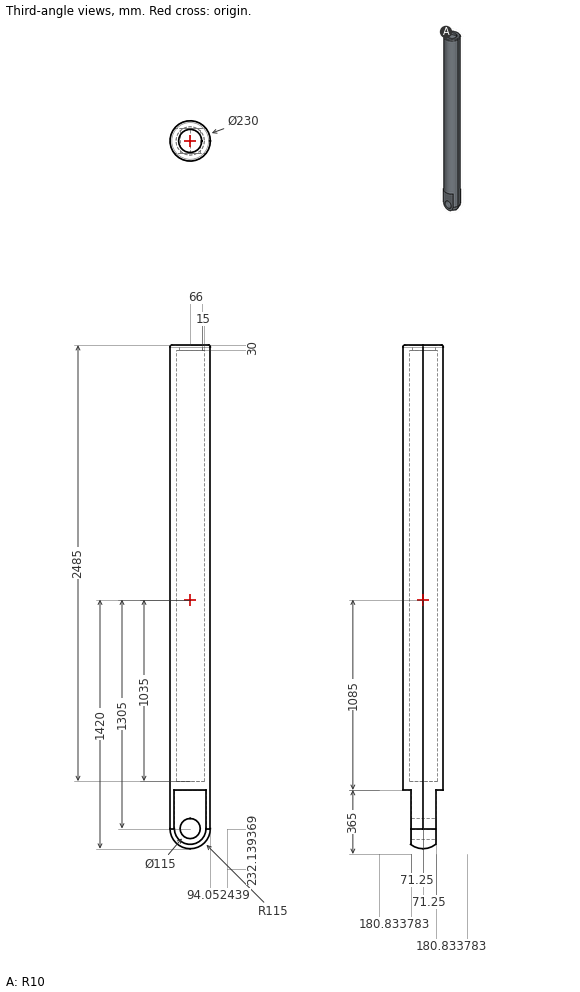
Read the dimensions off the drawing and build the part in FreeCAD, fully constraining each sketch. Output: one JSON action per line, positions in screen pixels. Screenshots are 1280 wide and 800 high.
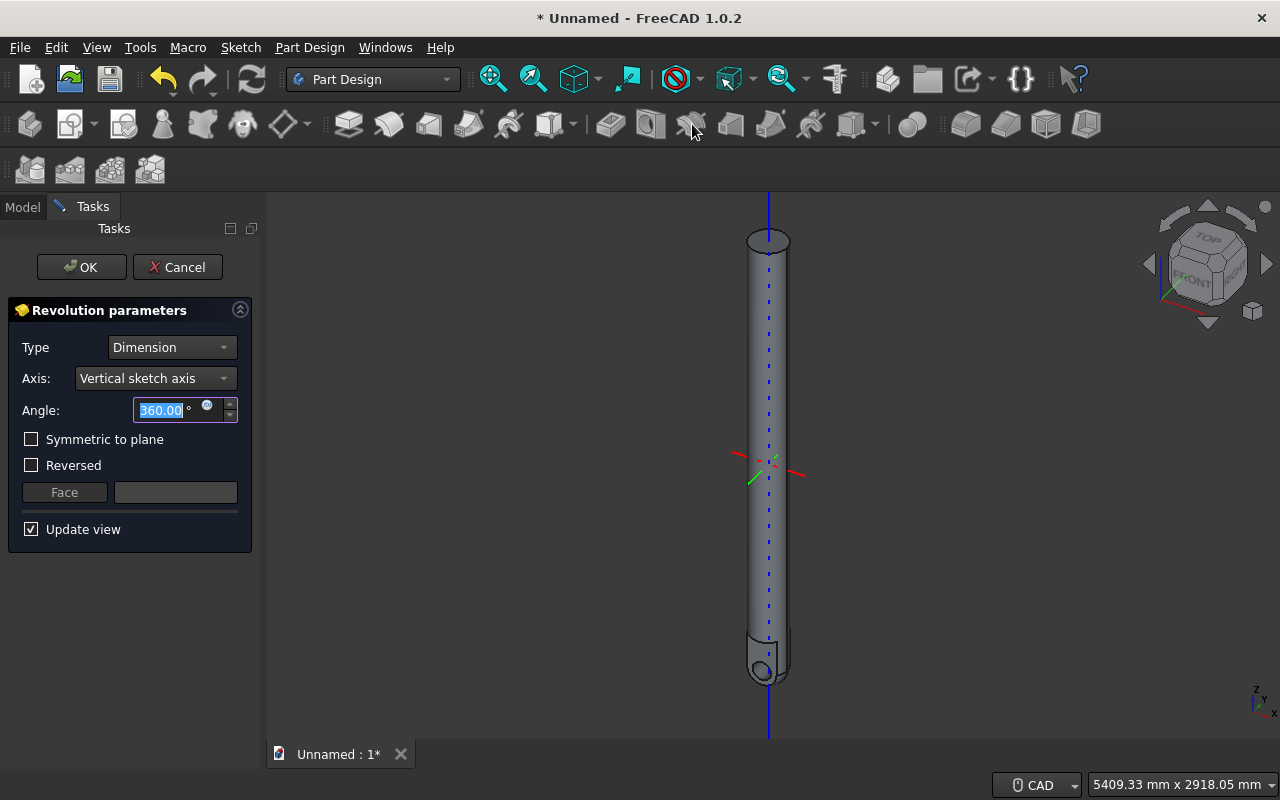
{"action": "left_click", "coordinate": [82, 267]}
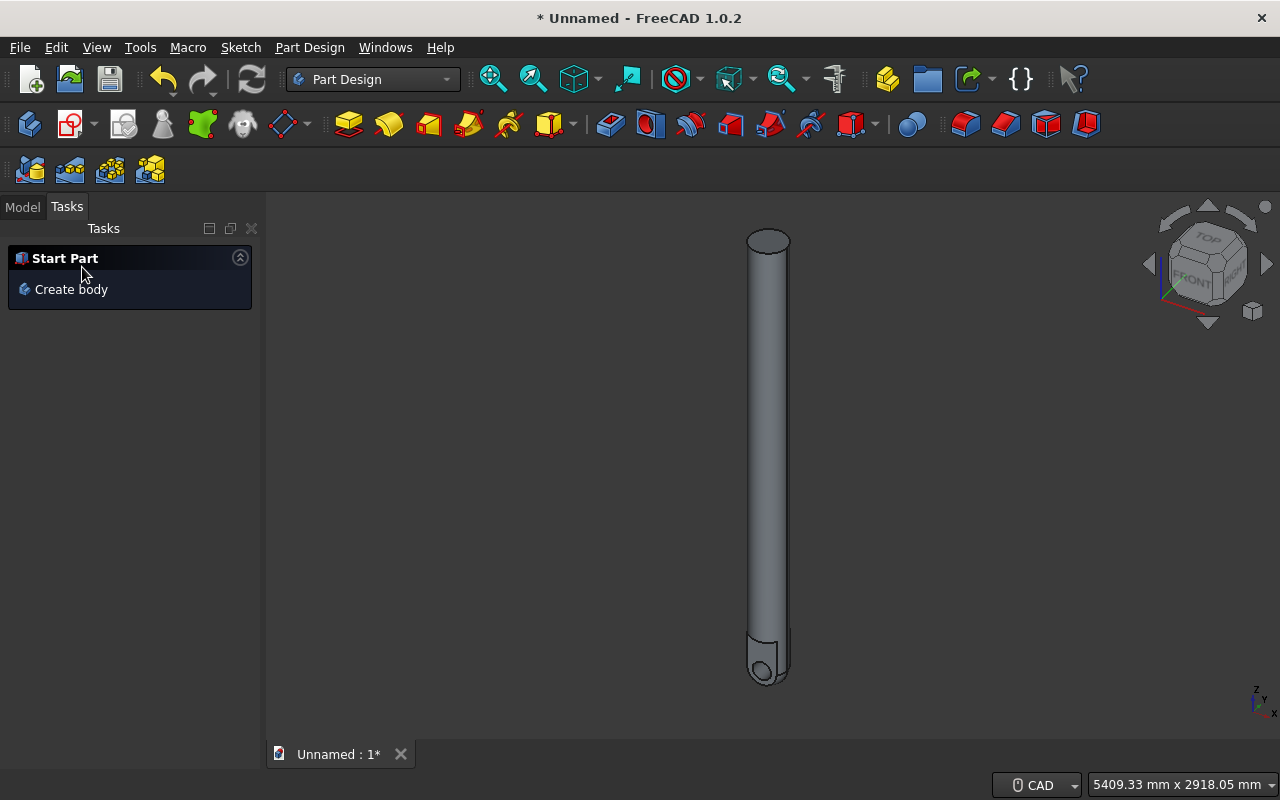
{"action": "left_click", "coordinate": [70, 124]}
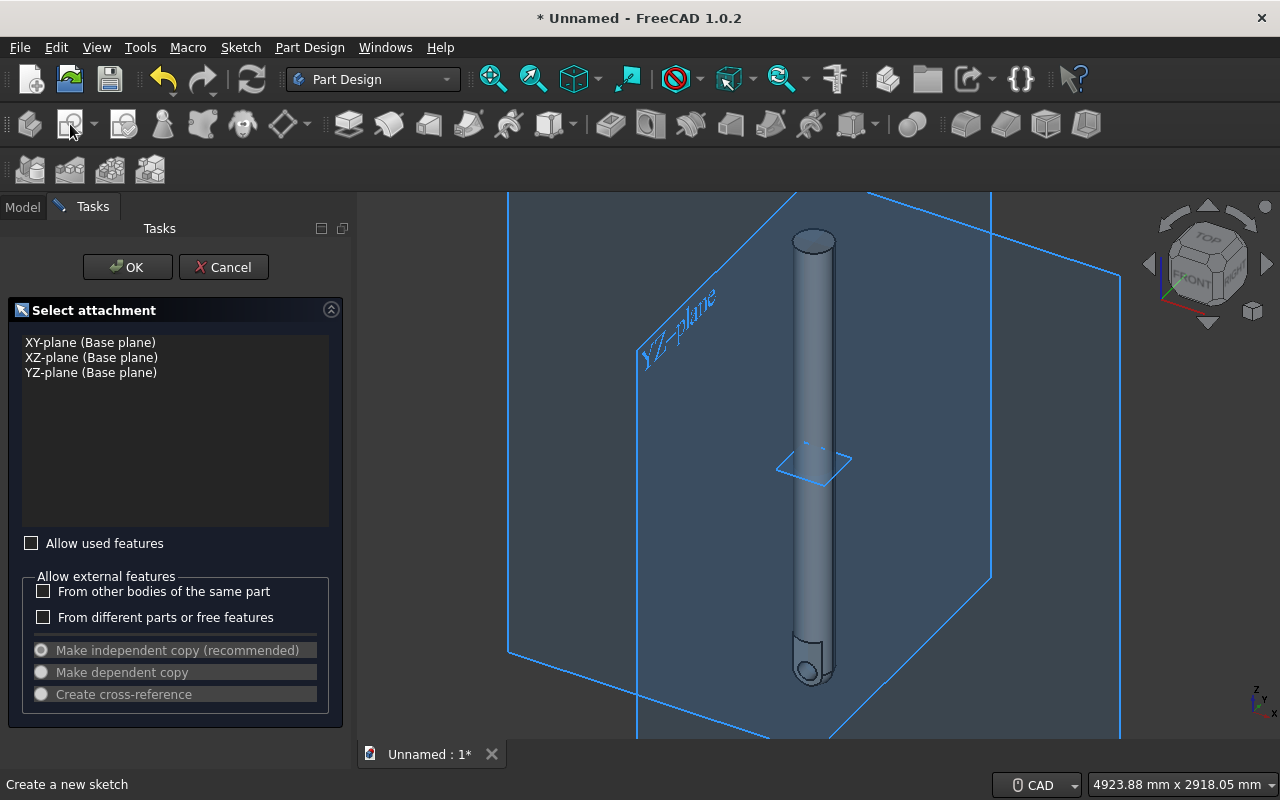
{"action": "left_click", "coordinate": [82, 358]}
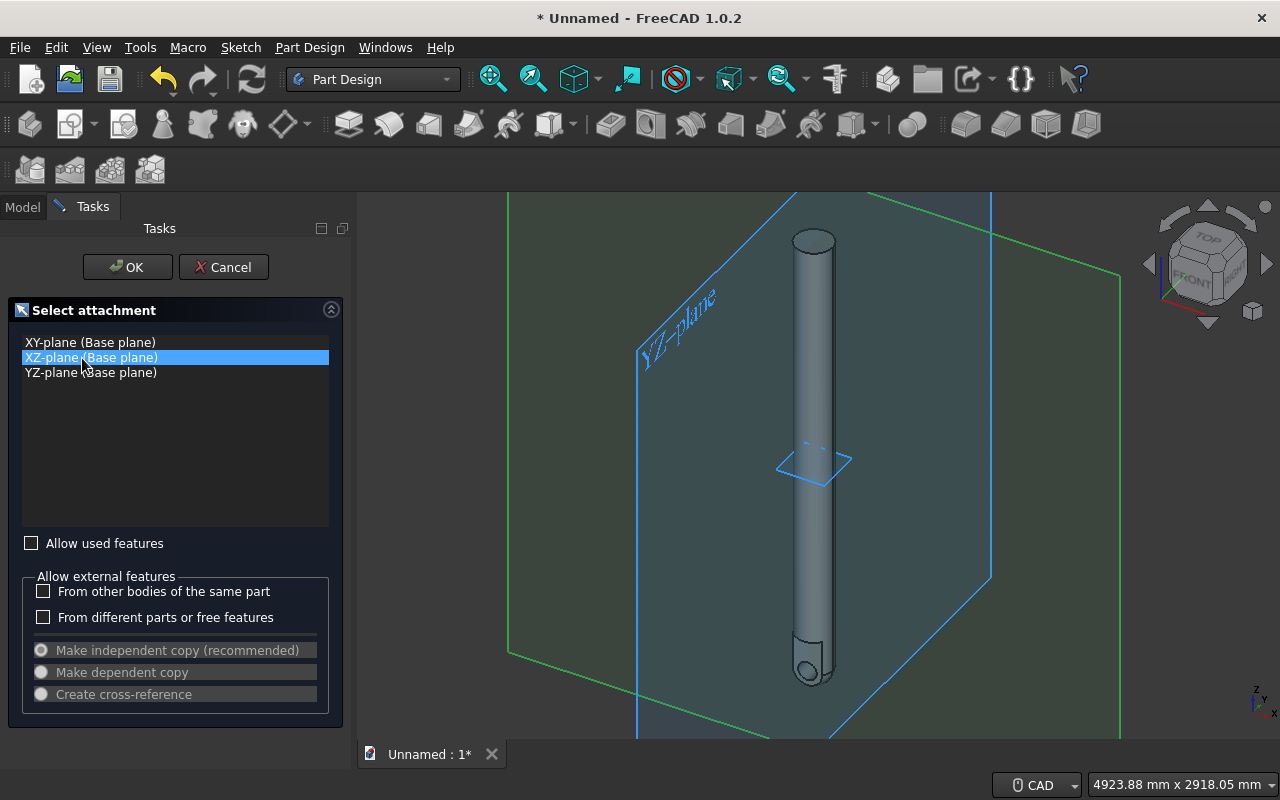
{"action": "left_click", "coordinate": [128, 267]}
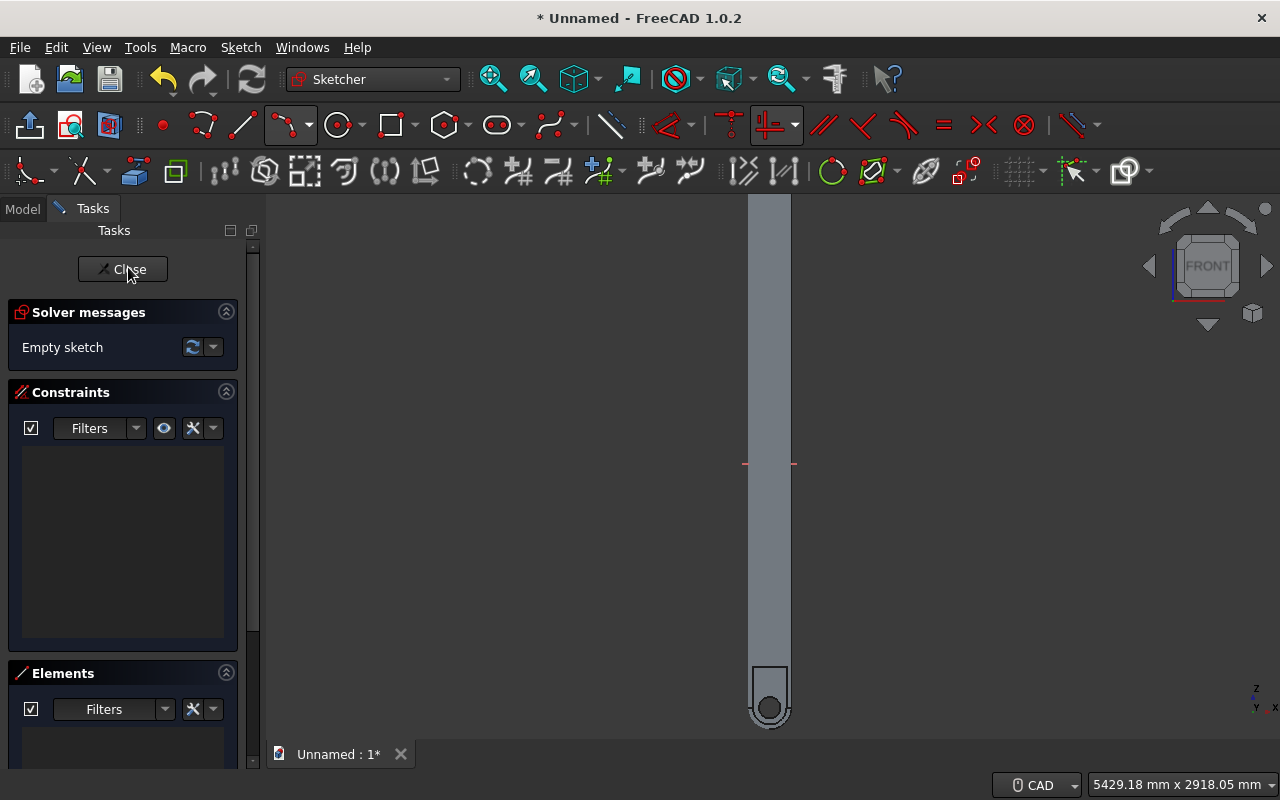
{"action": "key", "text": "q s"}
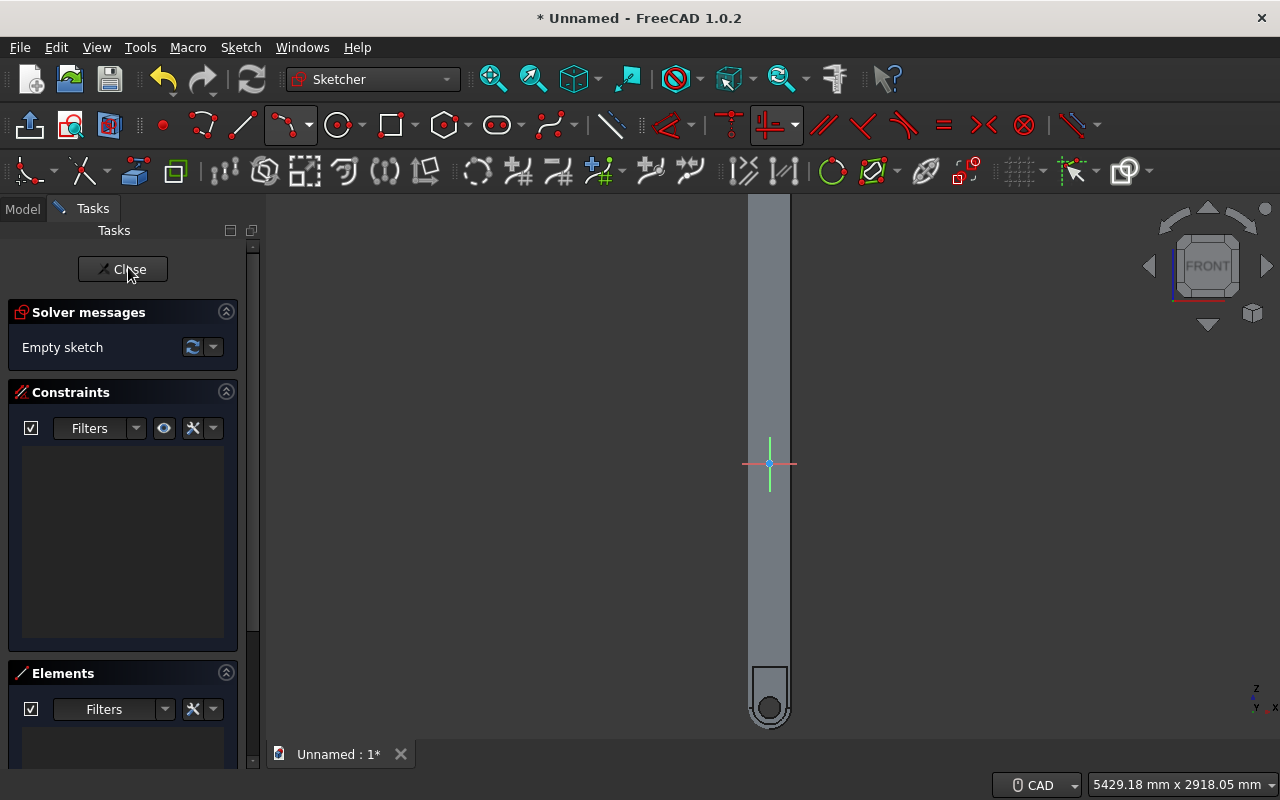
{"action": "scroll", "coordinate": [376, 653], "scroll_direction": "down", "scroll_amount": 1}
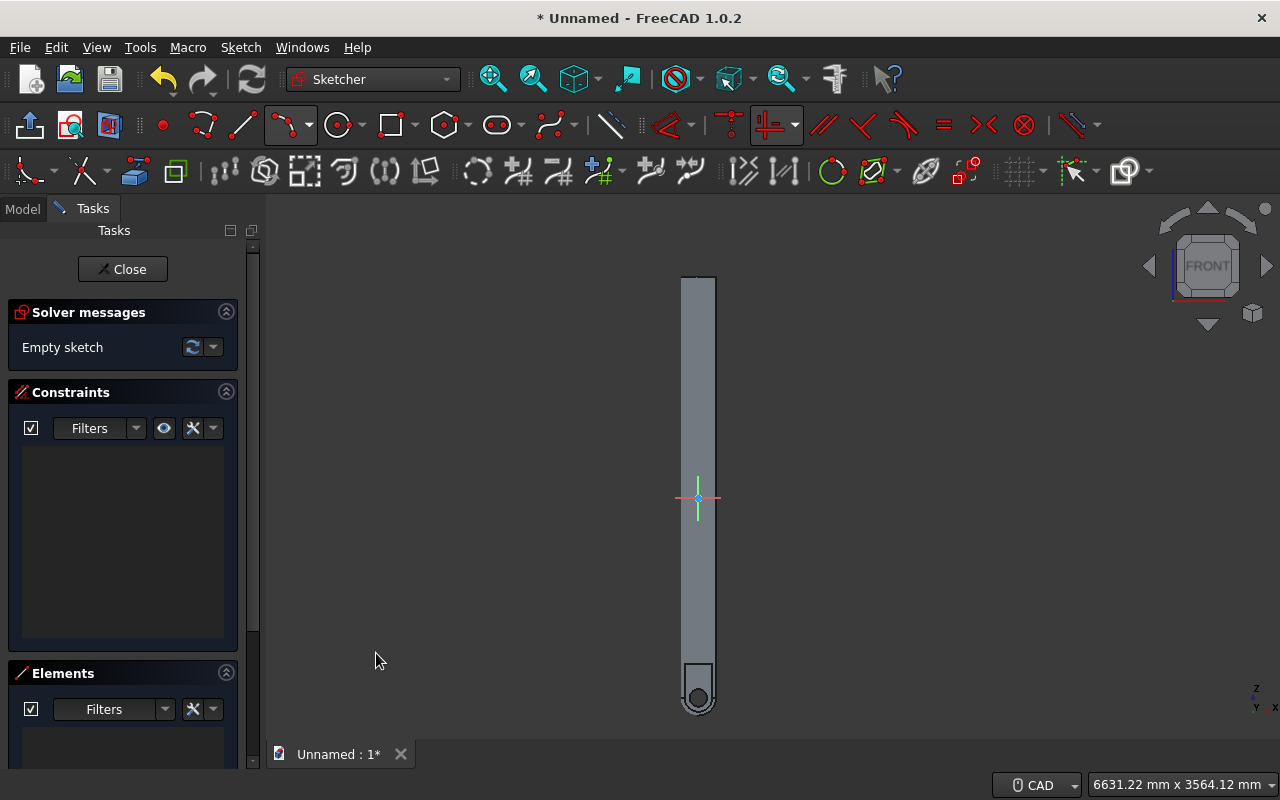
{"action": "left_click", "coordinate": [204, 126]}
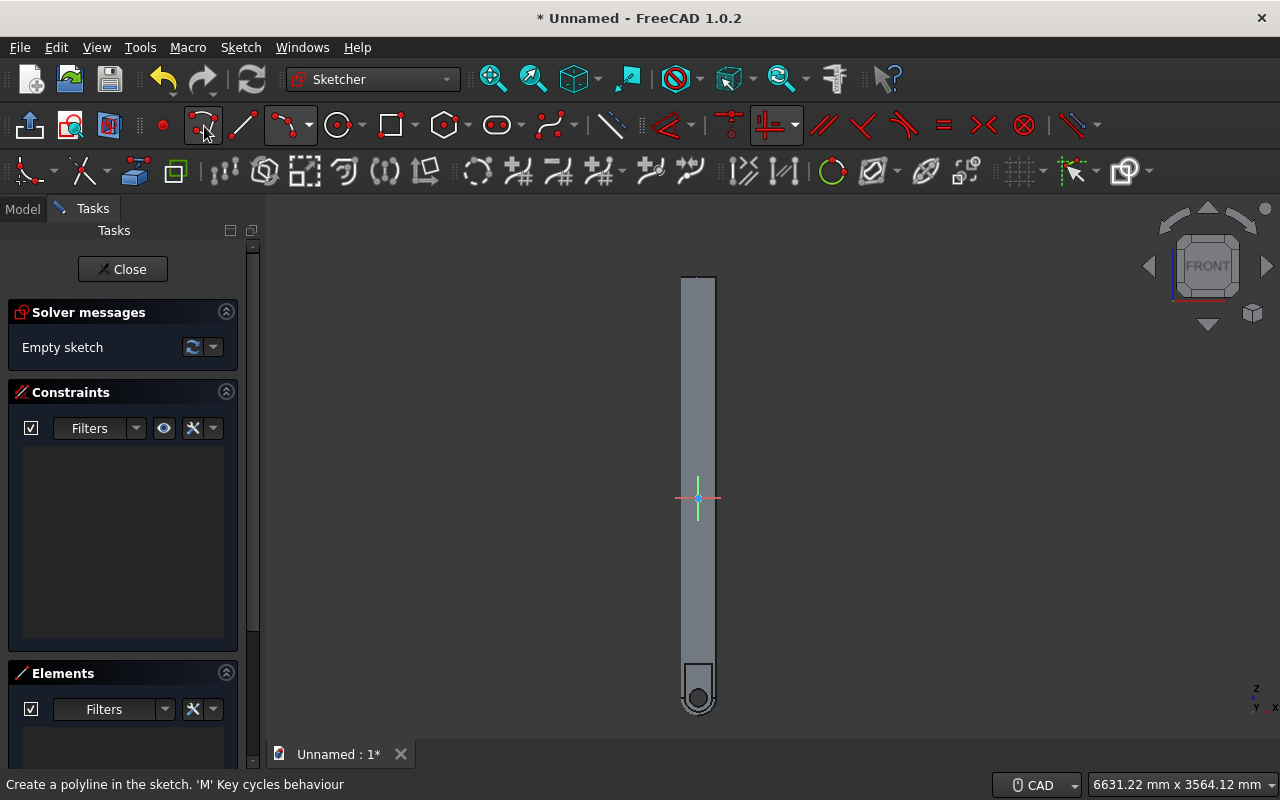
{"action": "left_click", "coordinate": [698, 657]}
{"action": "left_click", "coordinate": [707, 277]}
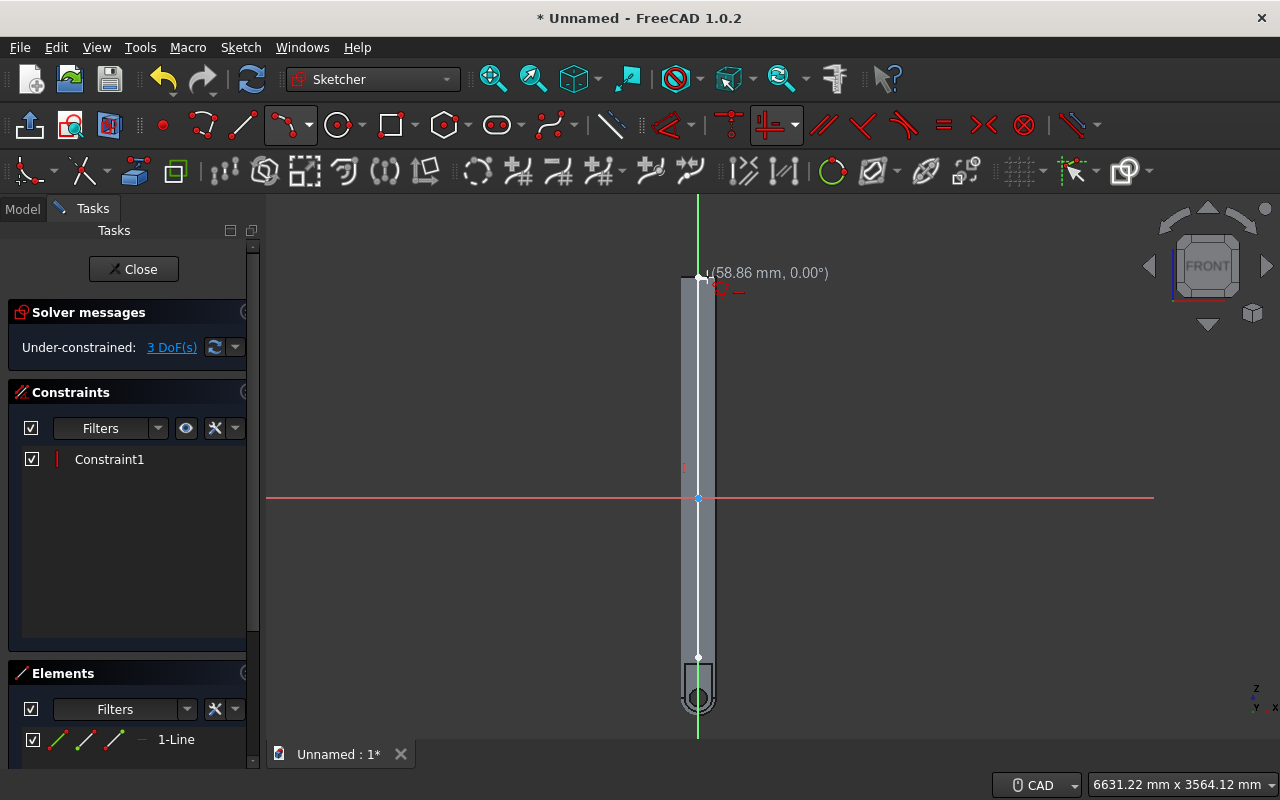
{"action": "scroll", "coordinate": [708, 277], "scroll_direction": "up", "scroll_amount": 3}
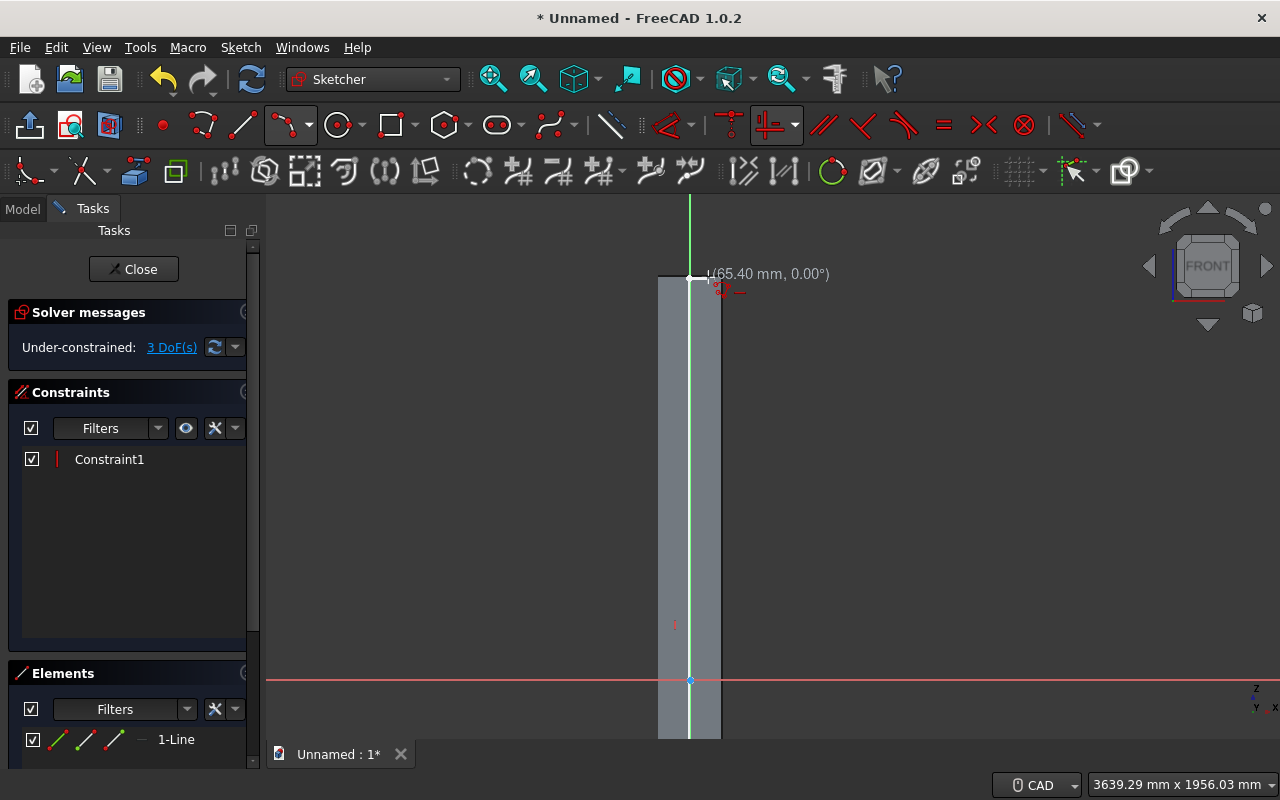
{"action": "left_click", "coordinate": [708, 277]}